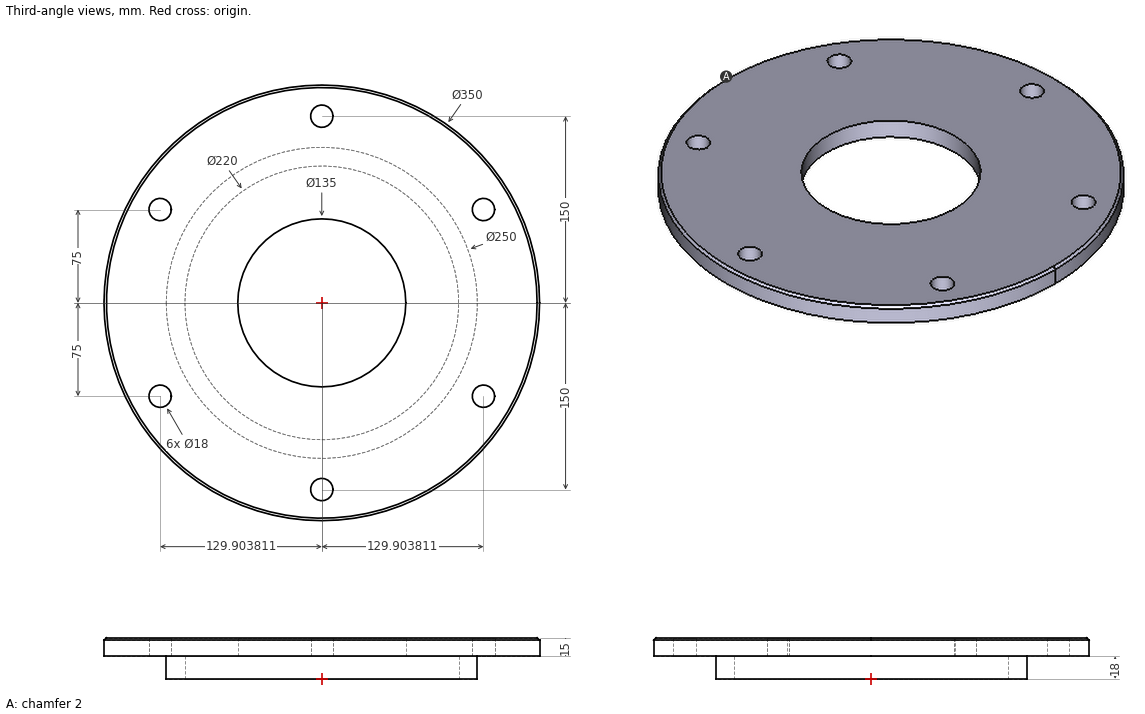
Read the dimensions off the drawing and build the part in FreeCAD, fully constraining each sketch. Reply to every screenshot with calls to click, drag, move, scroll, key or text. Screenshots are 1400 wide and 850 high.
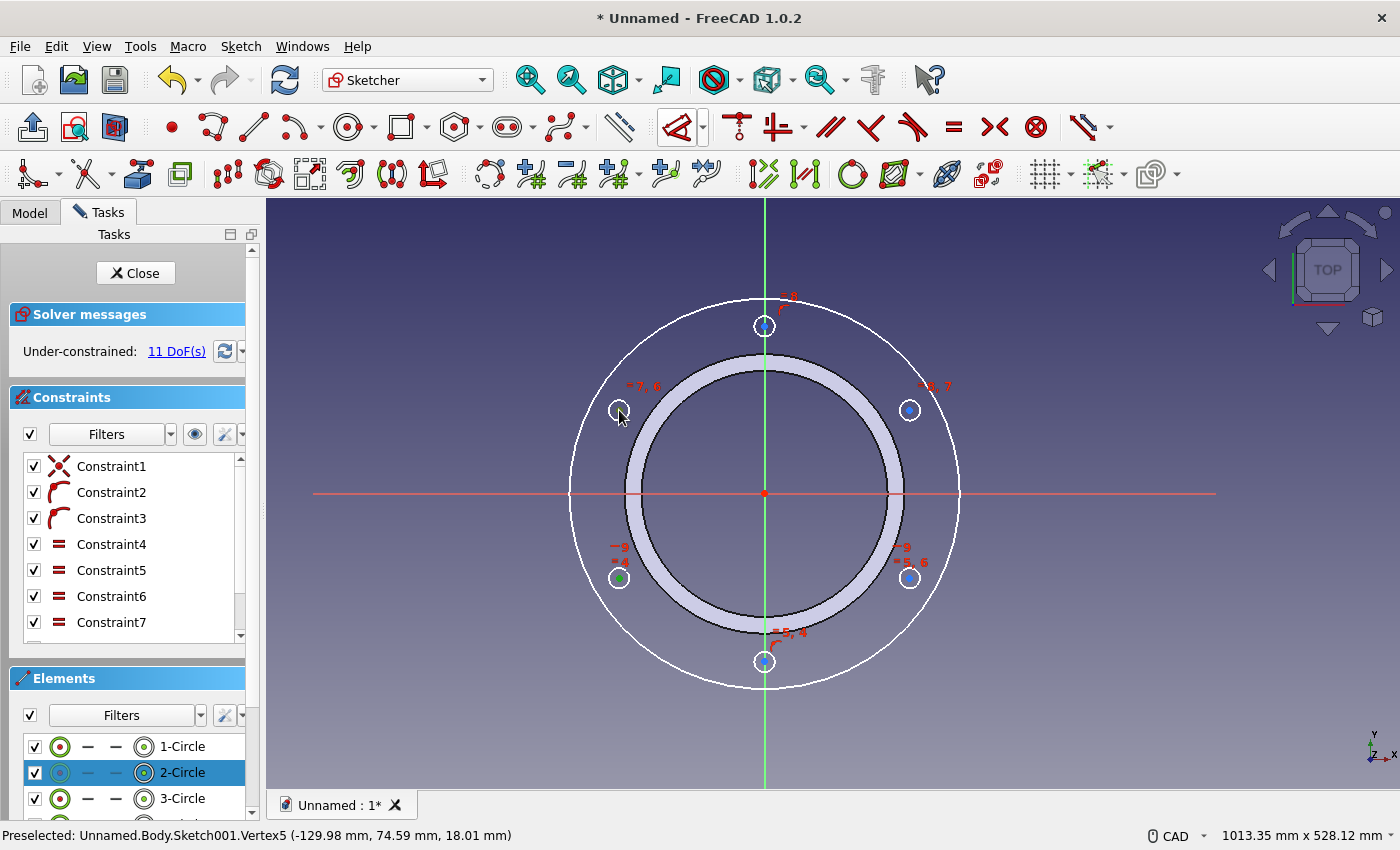
click(804, 128)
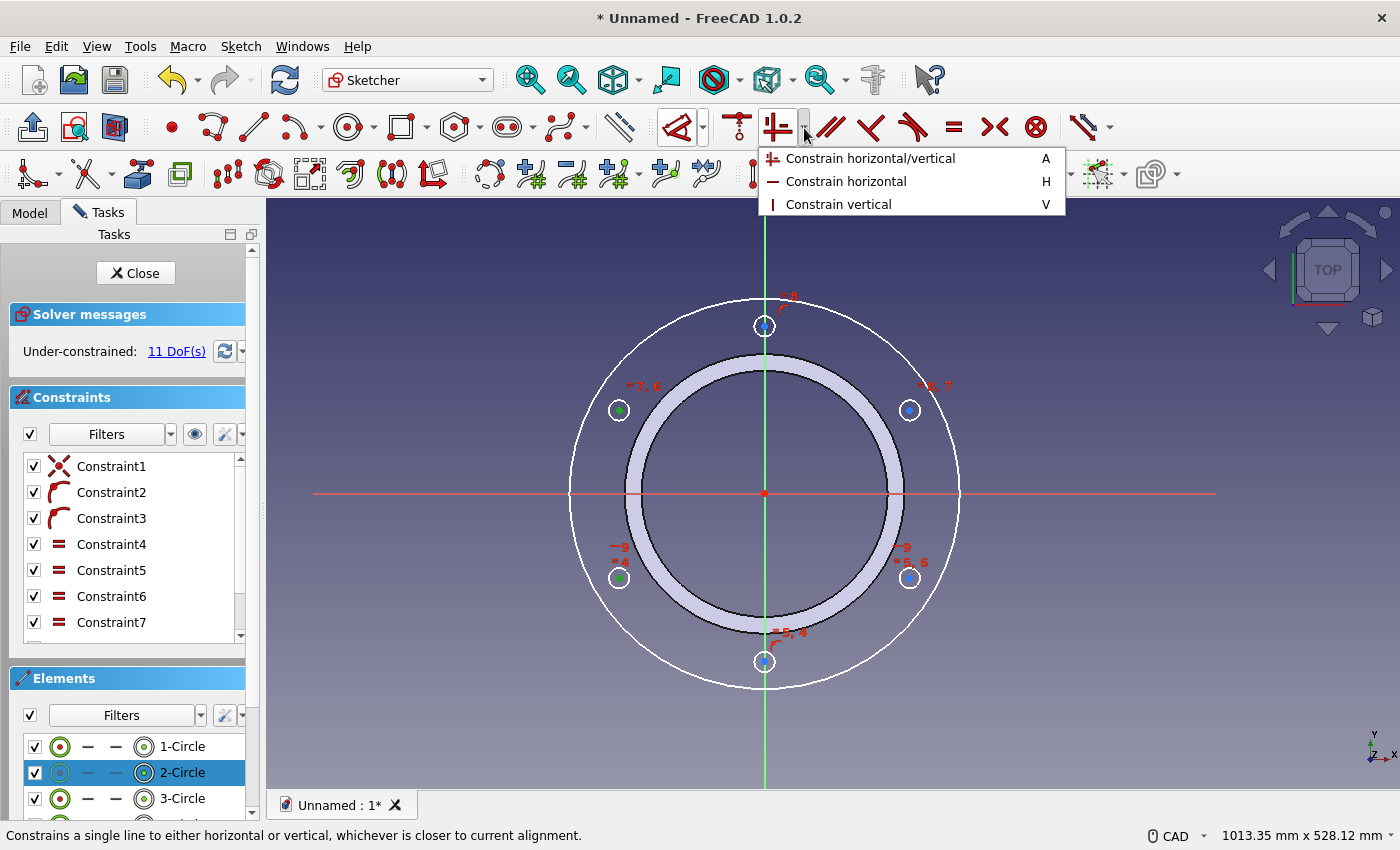
click(912, 204)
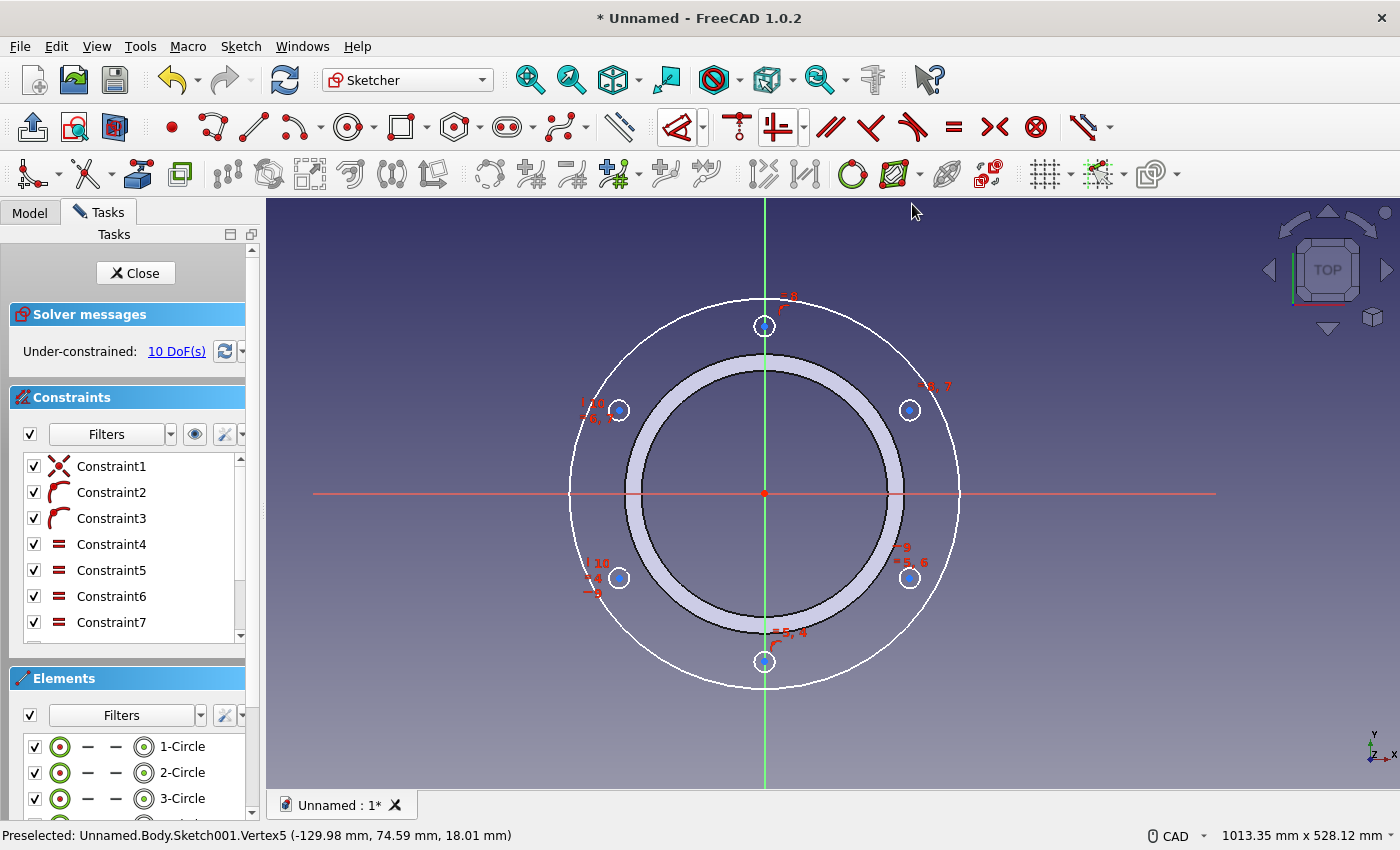
click(910, 578)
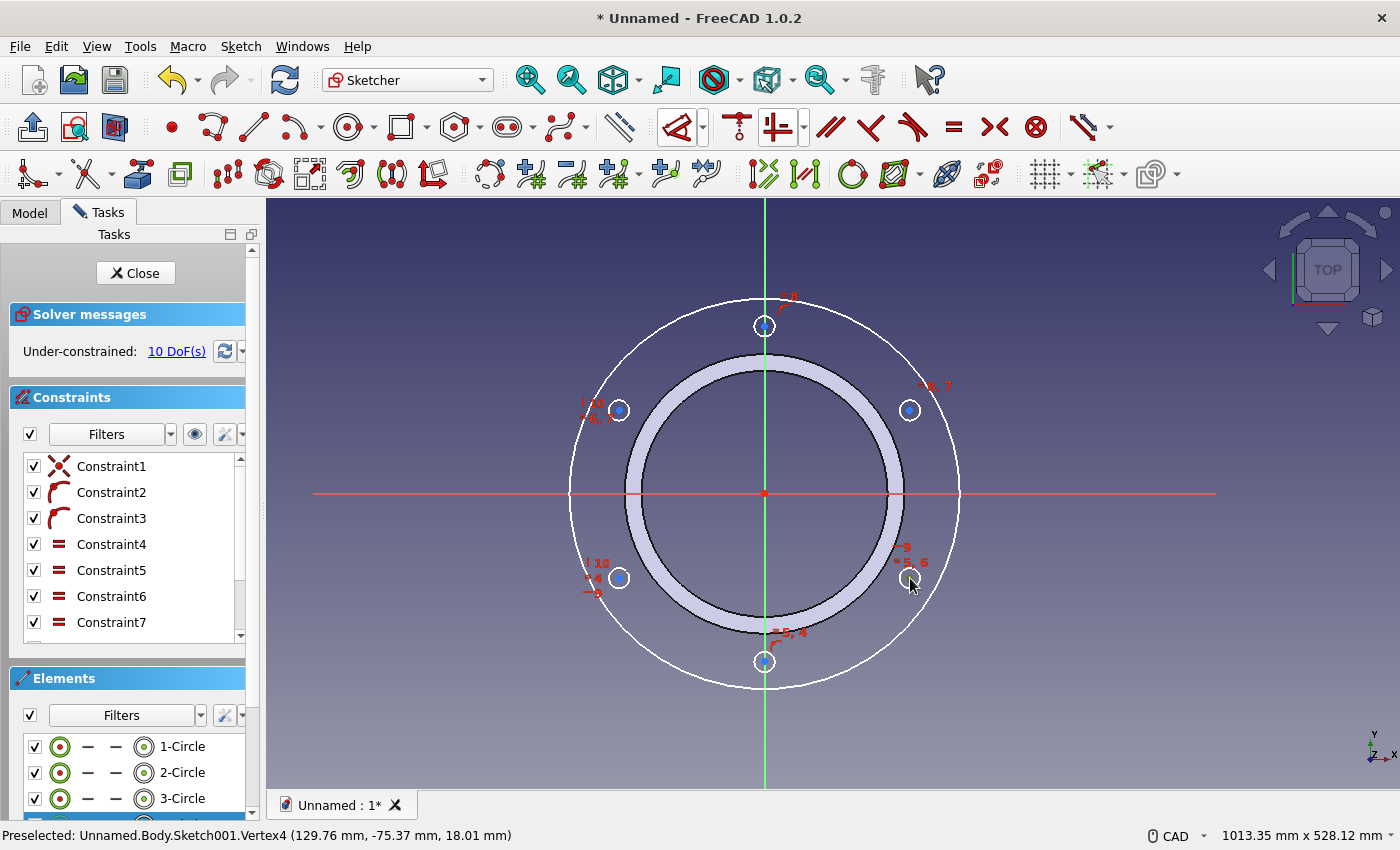
click(910, 410)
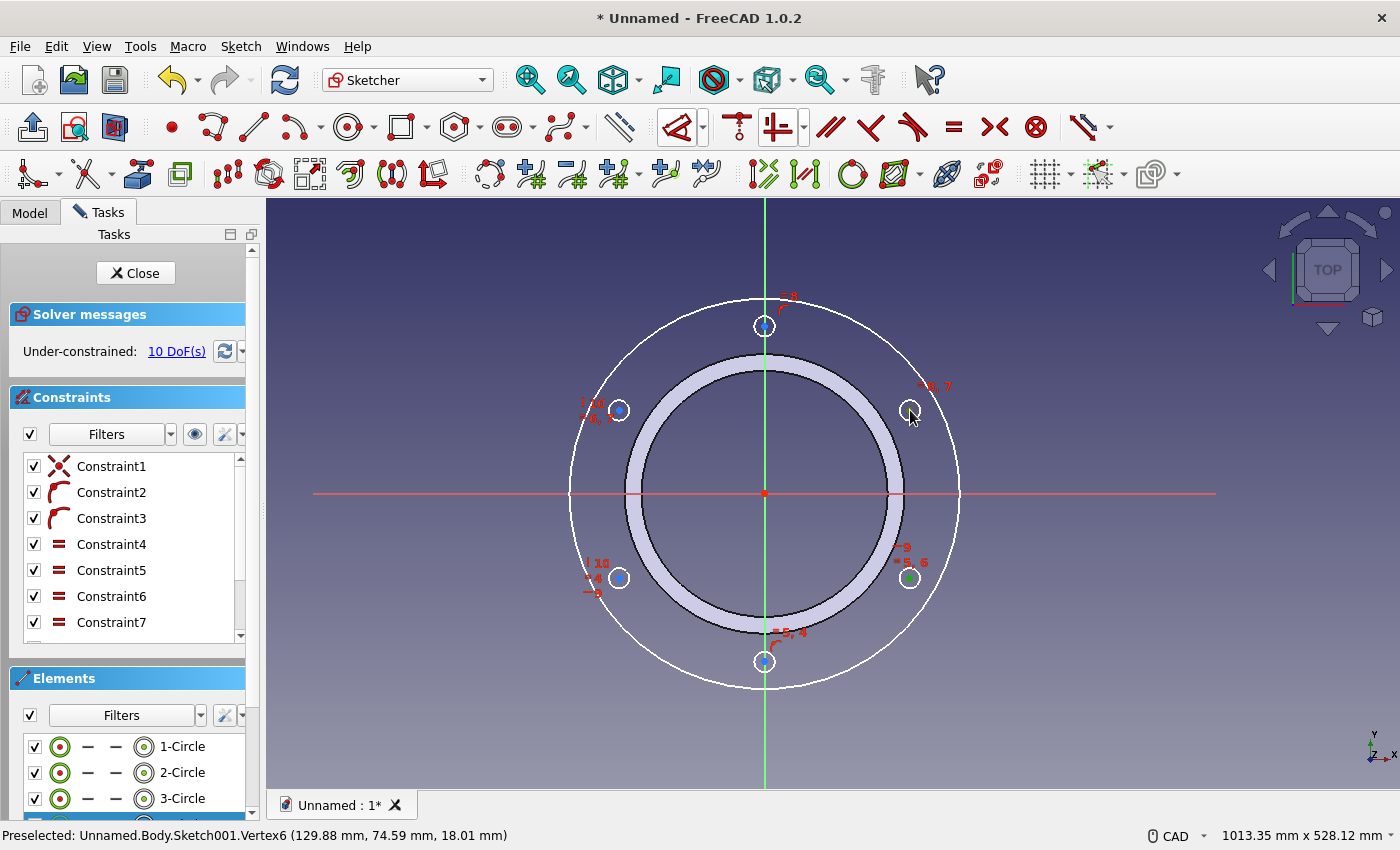
key(v)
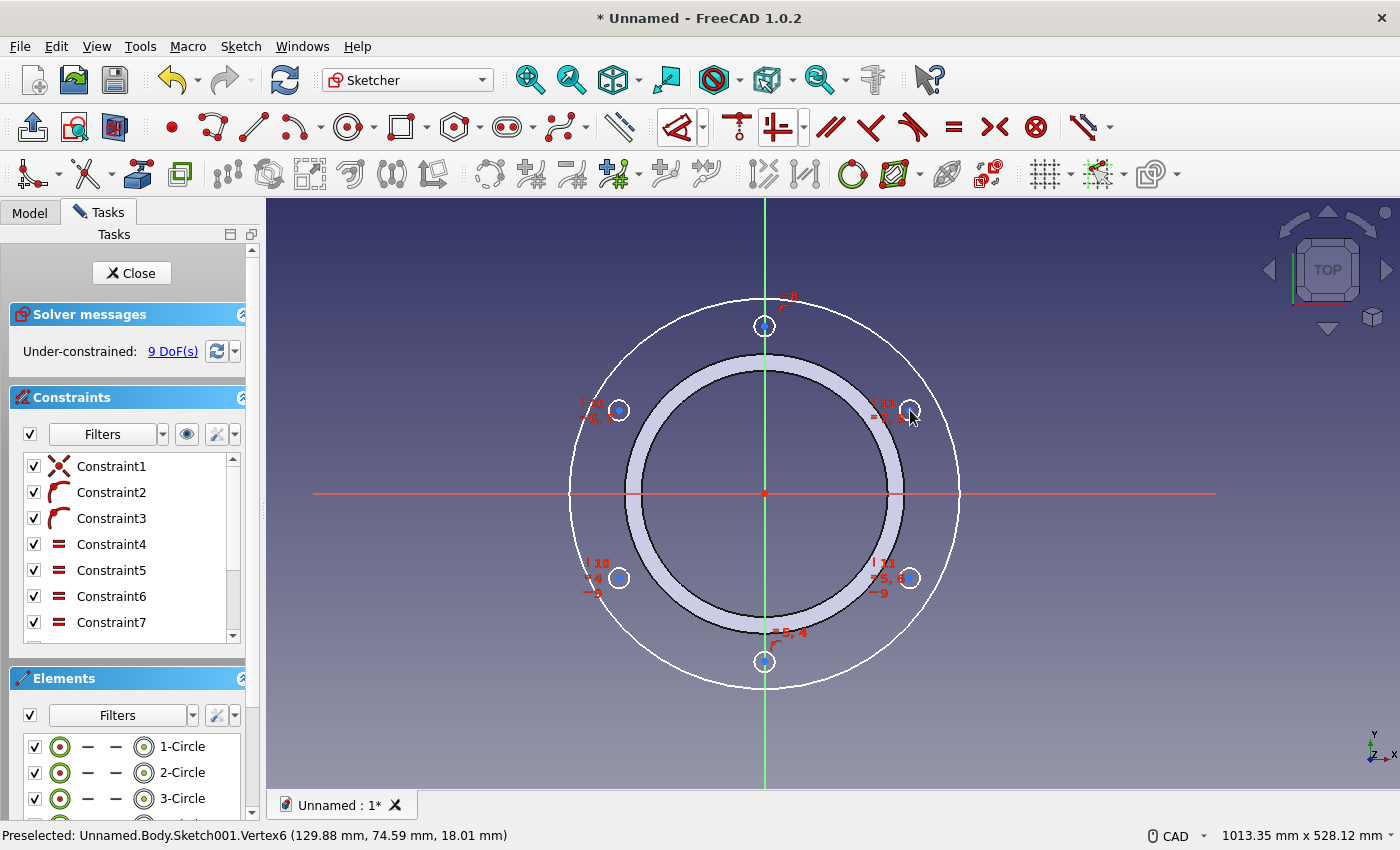
click(619, 410)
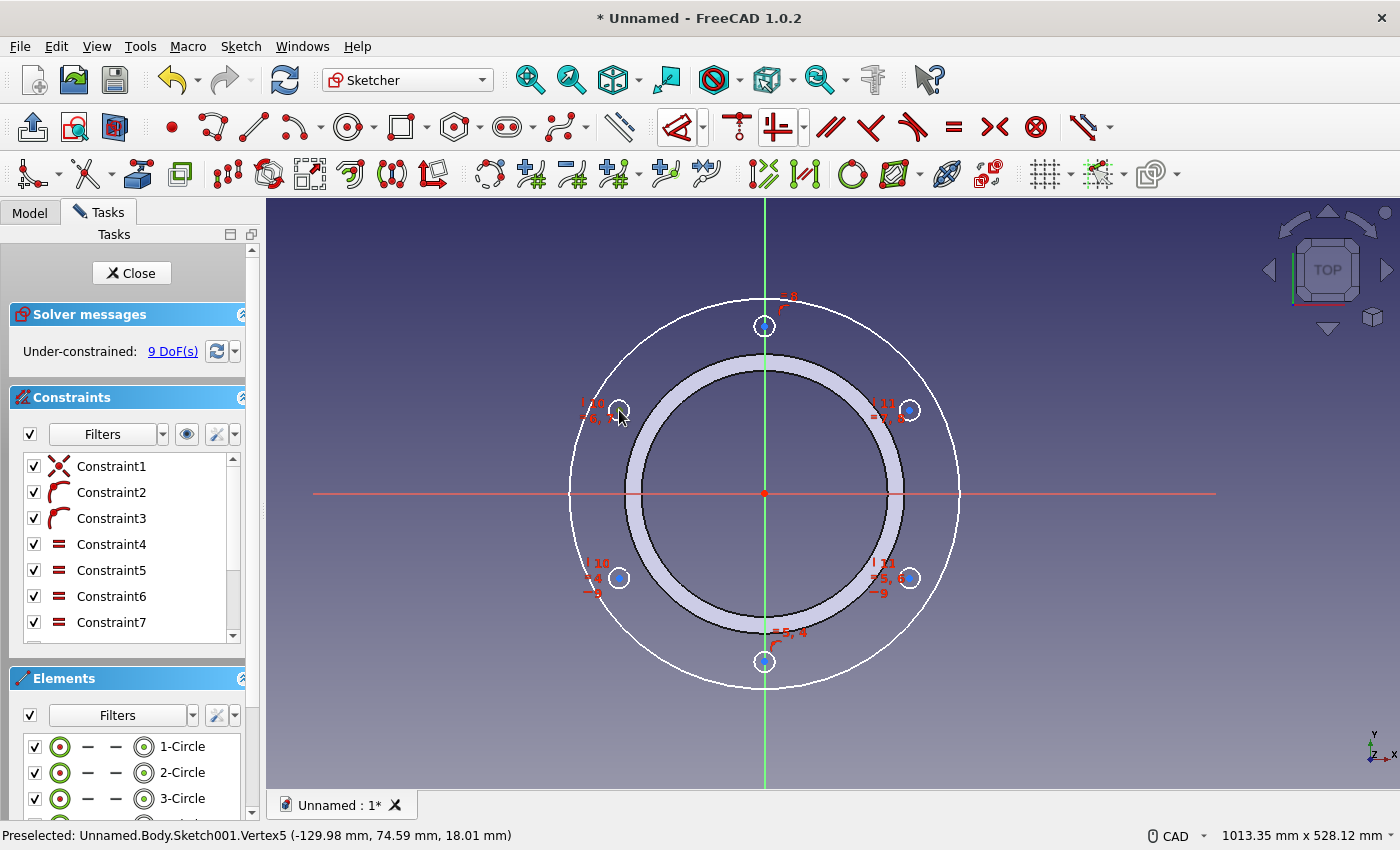
click(910, 410)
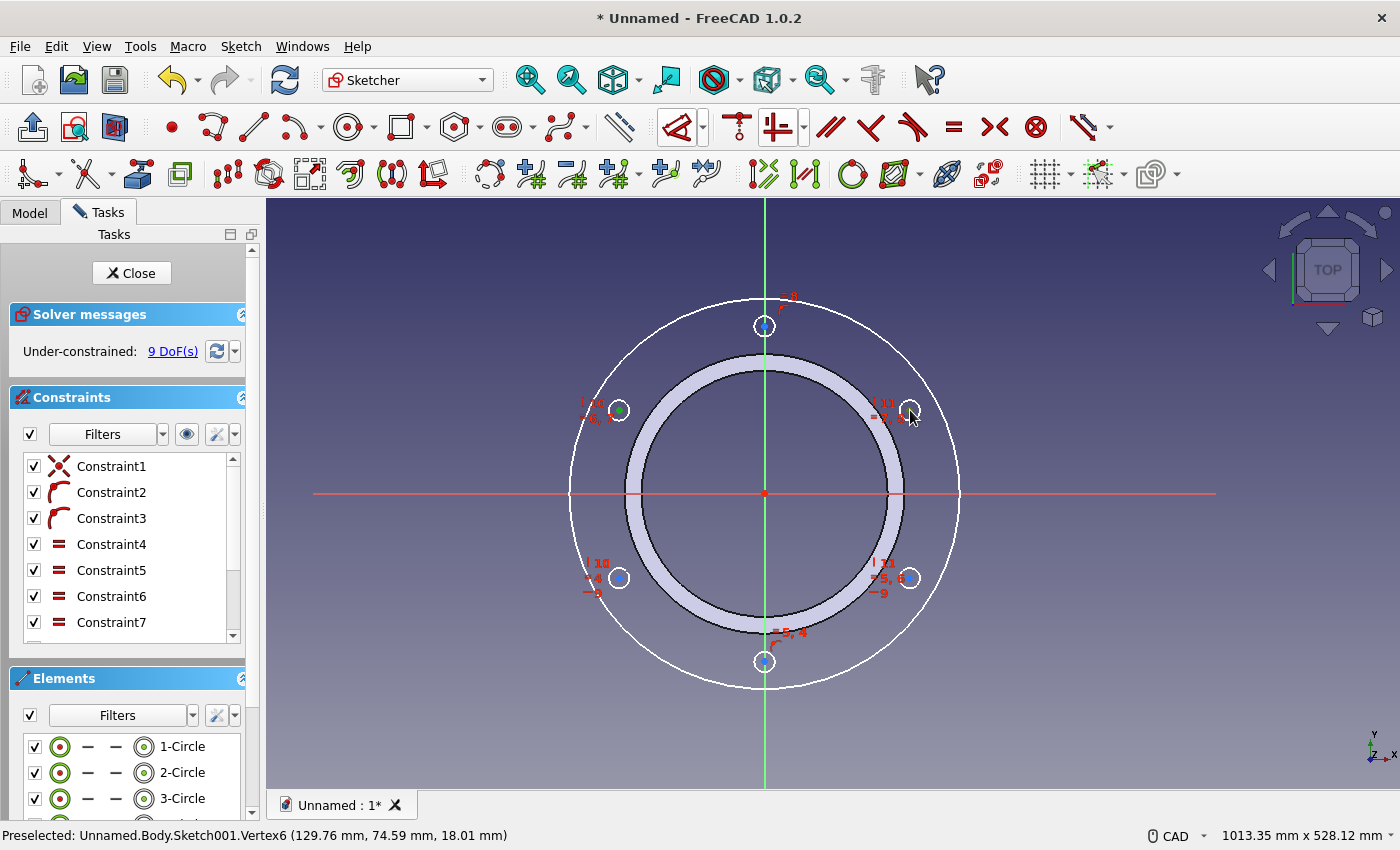
key(h)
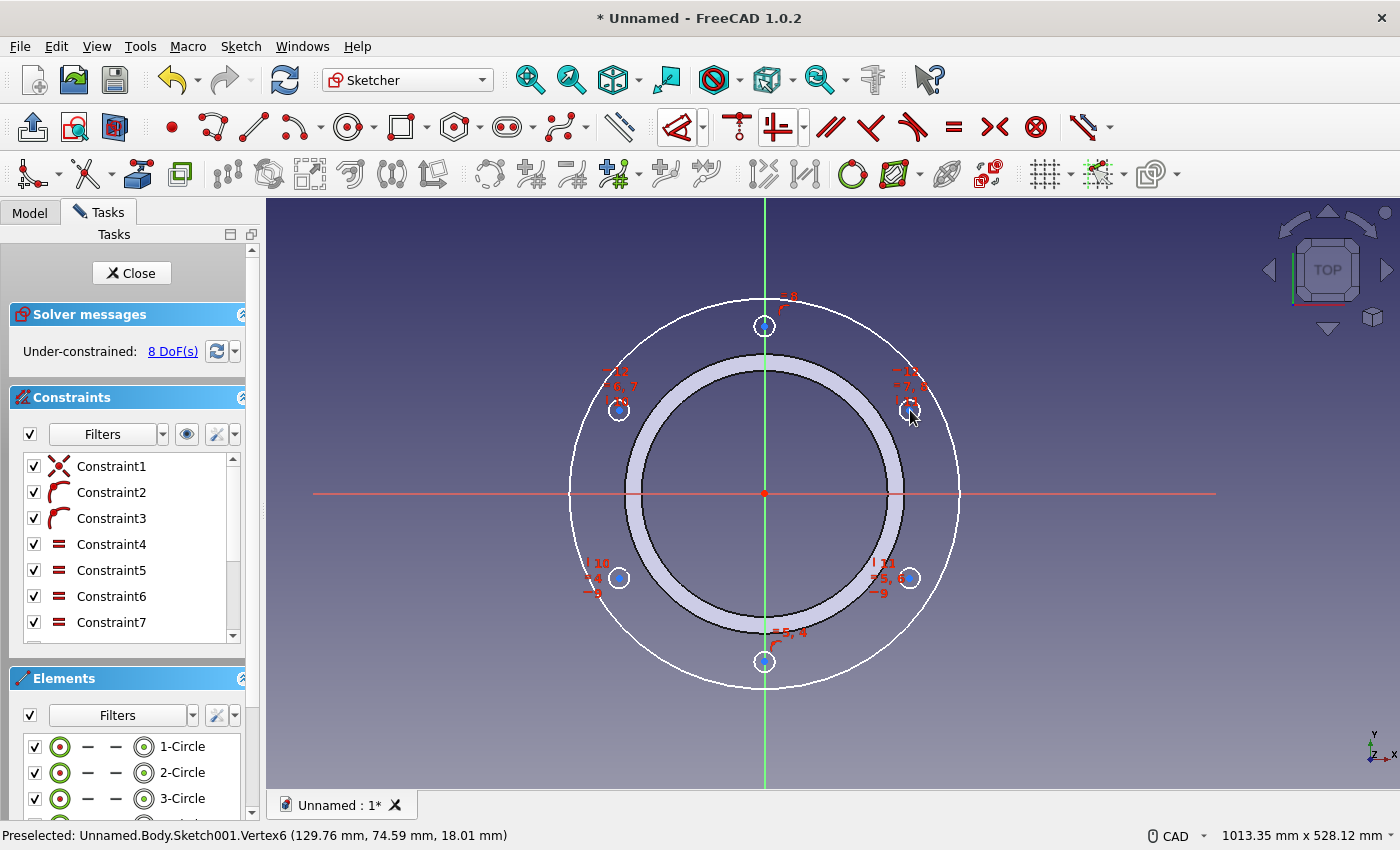
click(902, 355)